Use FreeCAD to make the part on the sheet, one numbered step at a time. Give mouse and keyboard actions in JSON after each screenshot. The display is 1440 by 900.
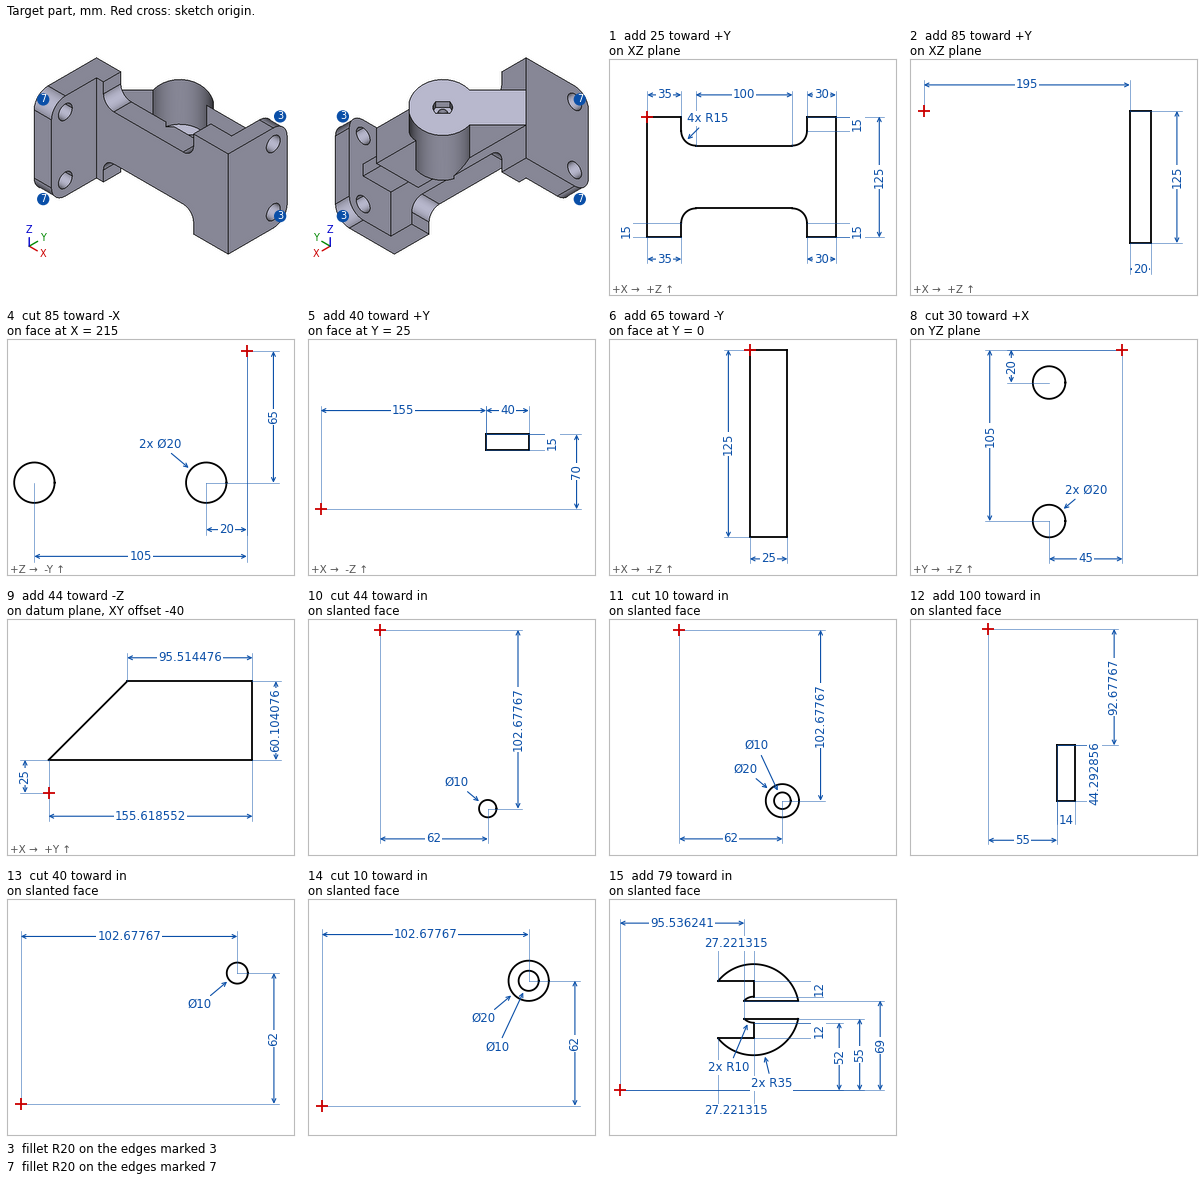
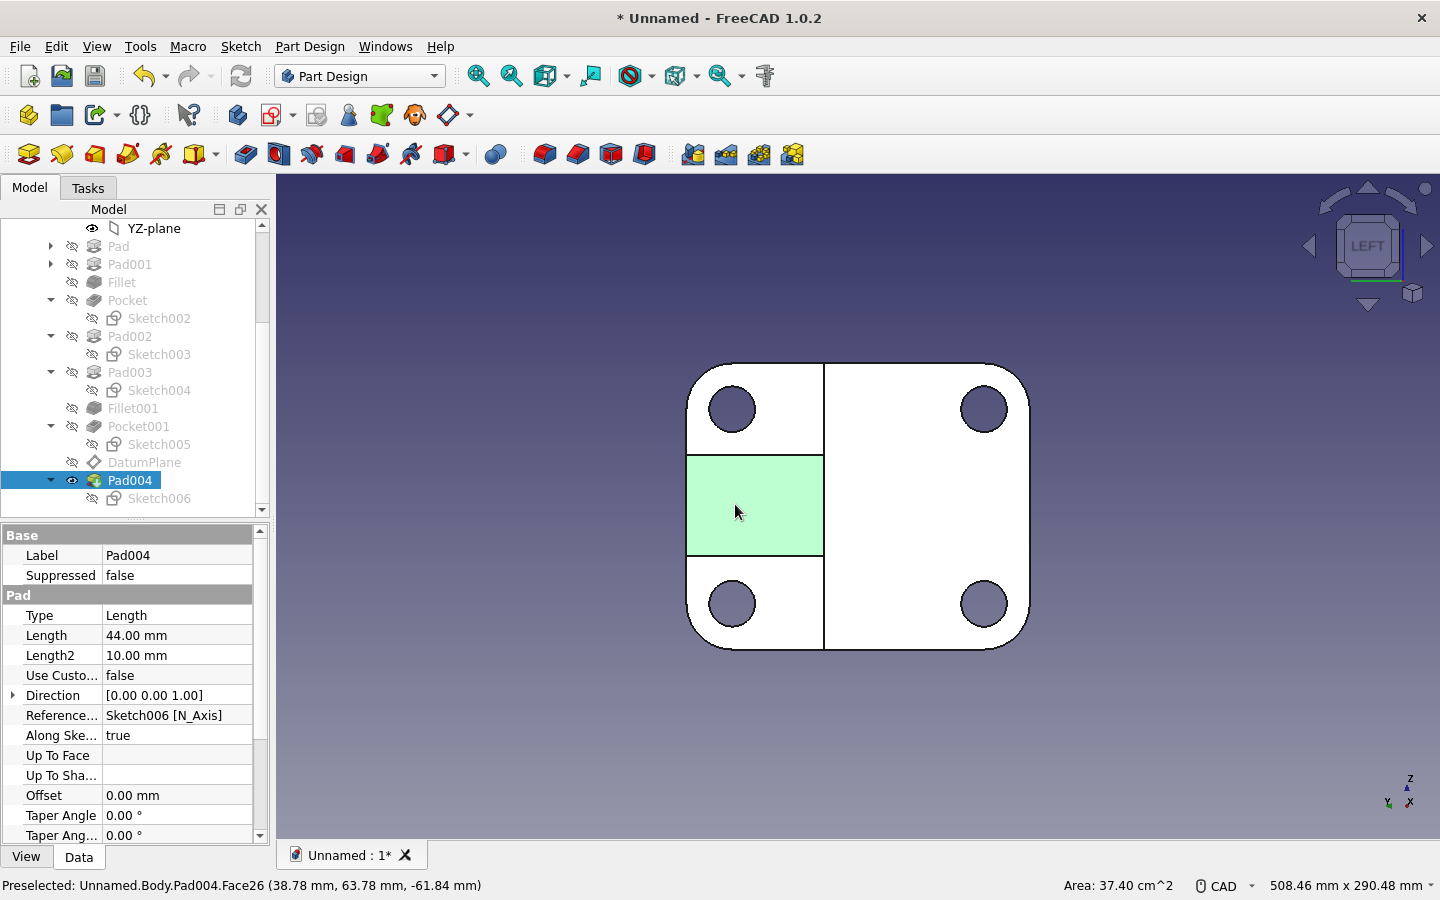
{"action": "left_click", "coordinate": [270, 116]}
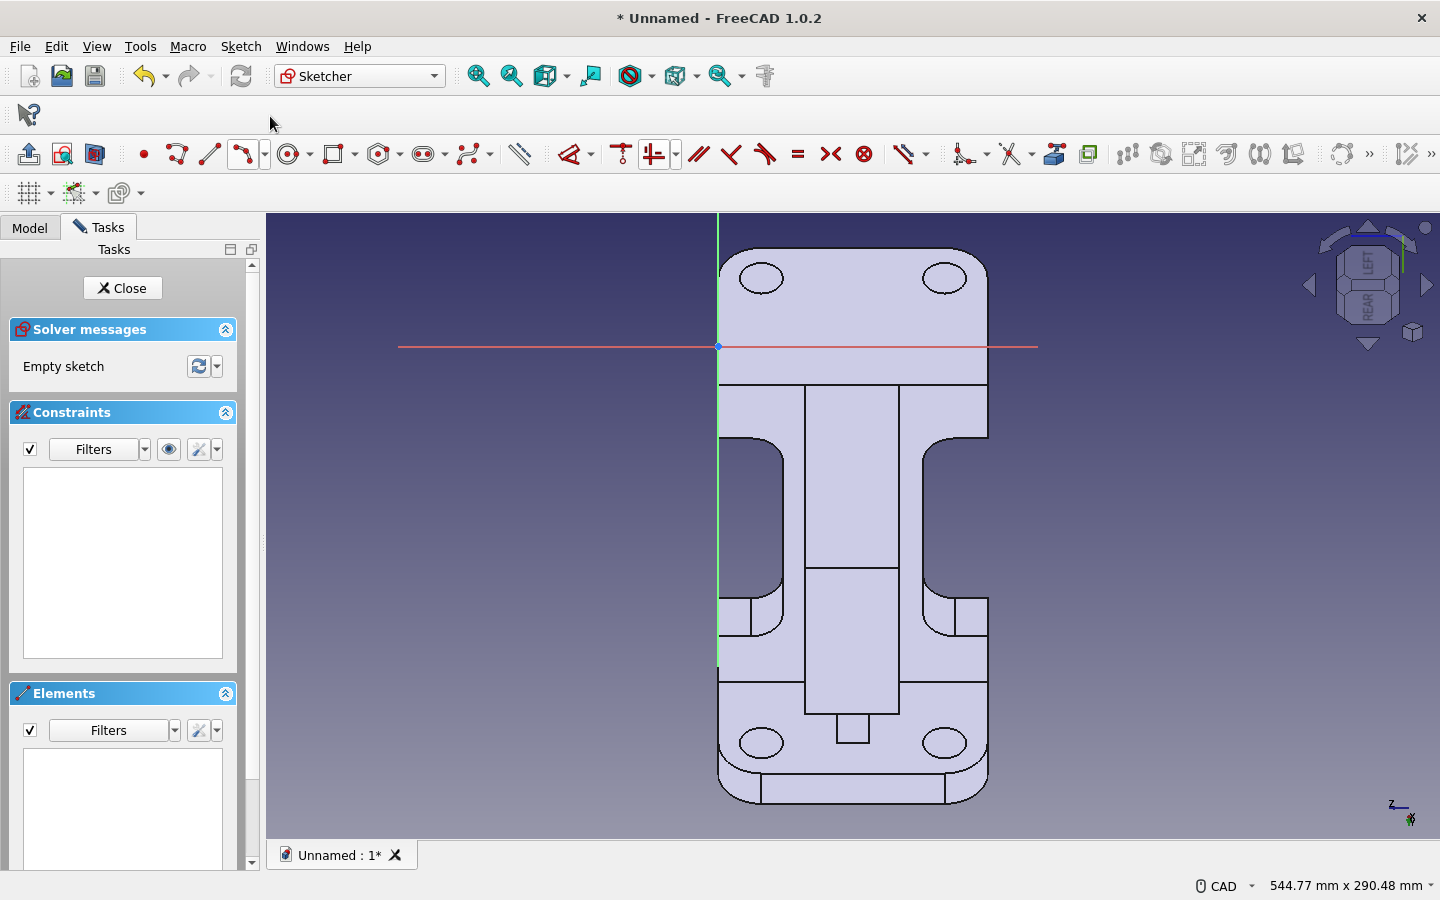
{"action": "scroll", "coordinate": [855, 570], "scroll_direction": "up", "scroll_amount": 15}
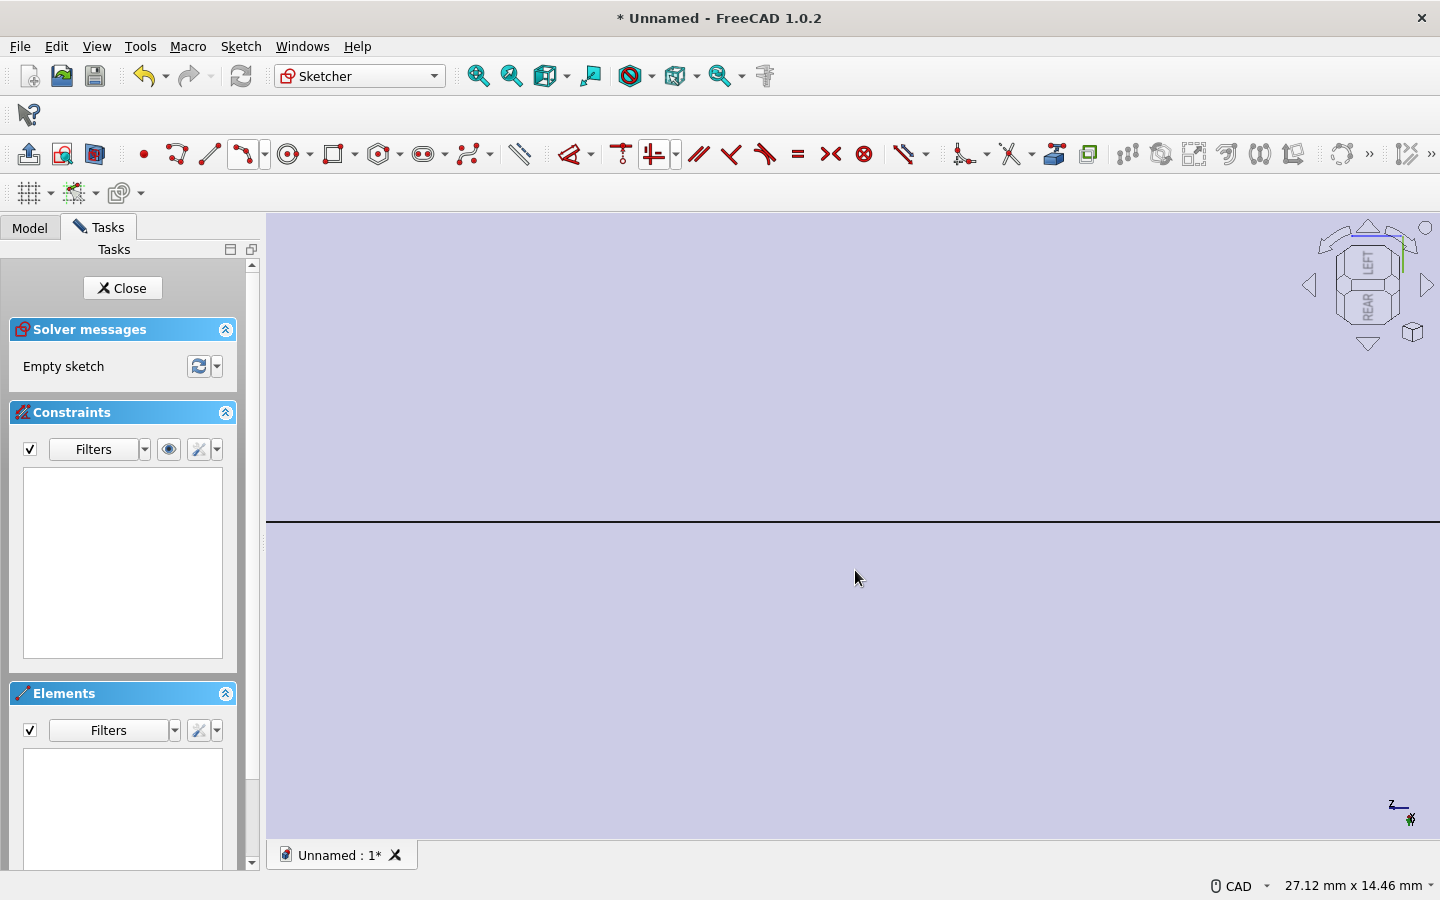
{"action": "left_click", "coordinate": [288, 154]}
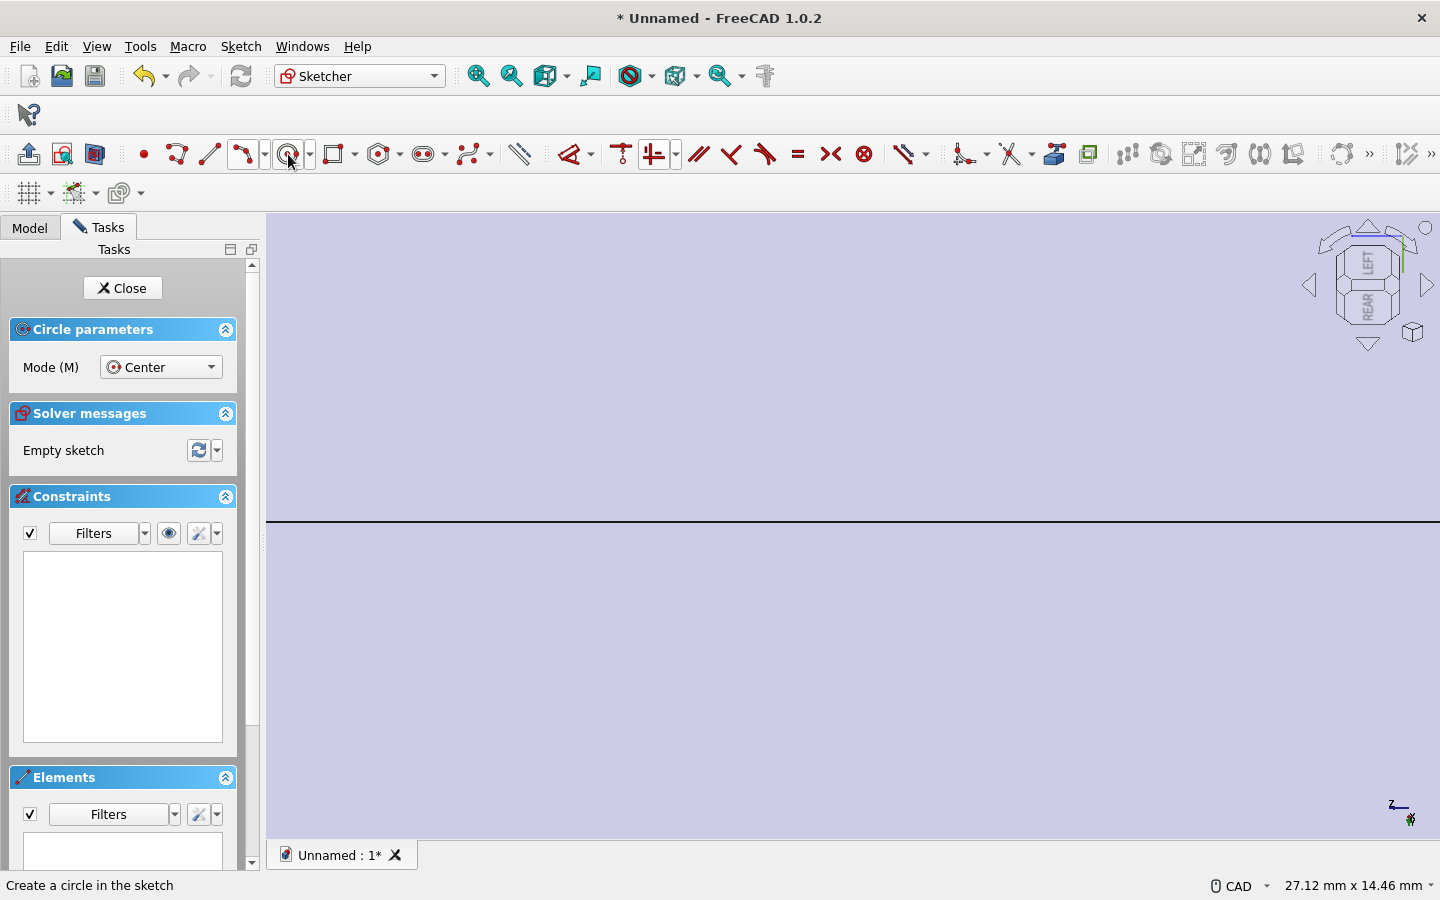
{"action": "left_click", "coordinate": [784, 522]}
{"action": "left_click", "coordinate": [937, 369]}
{"action": "key", "text": "Escape"}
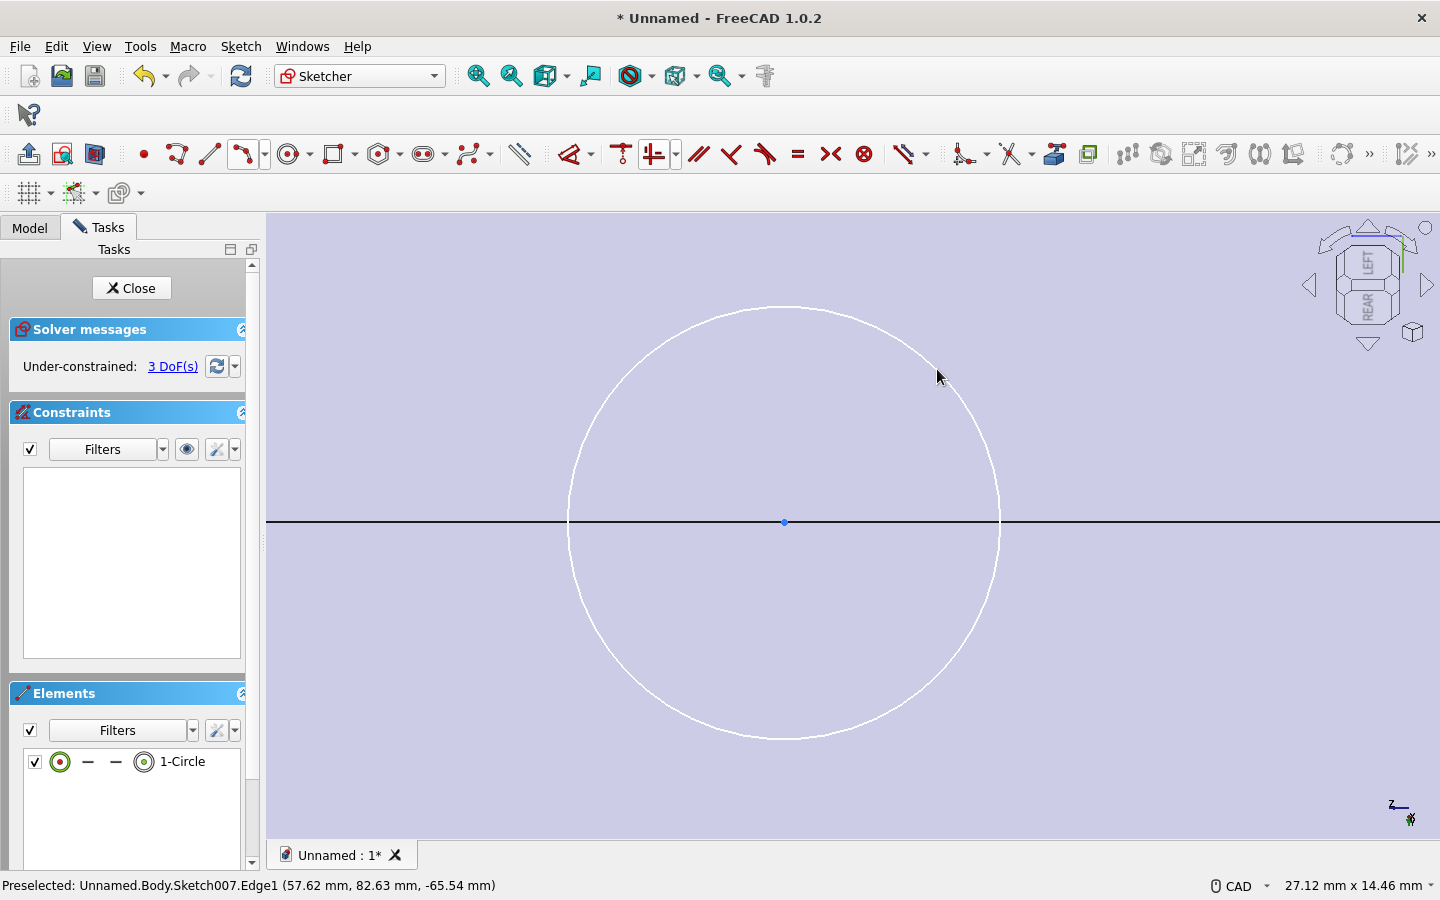
{"action": "left_click", "coordinate": [568, 154]}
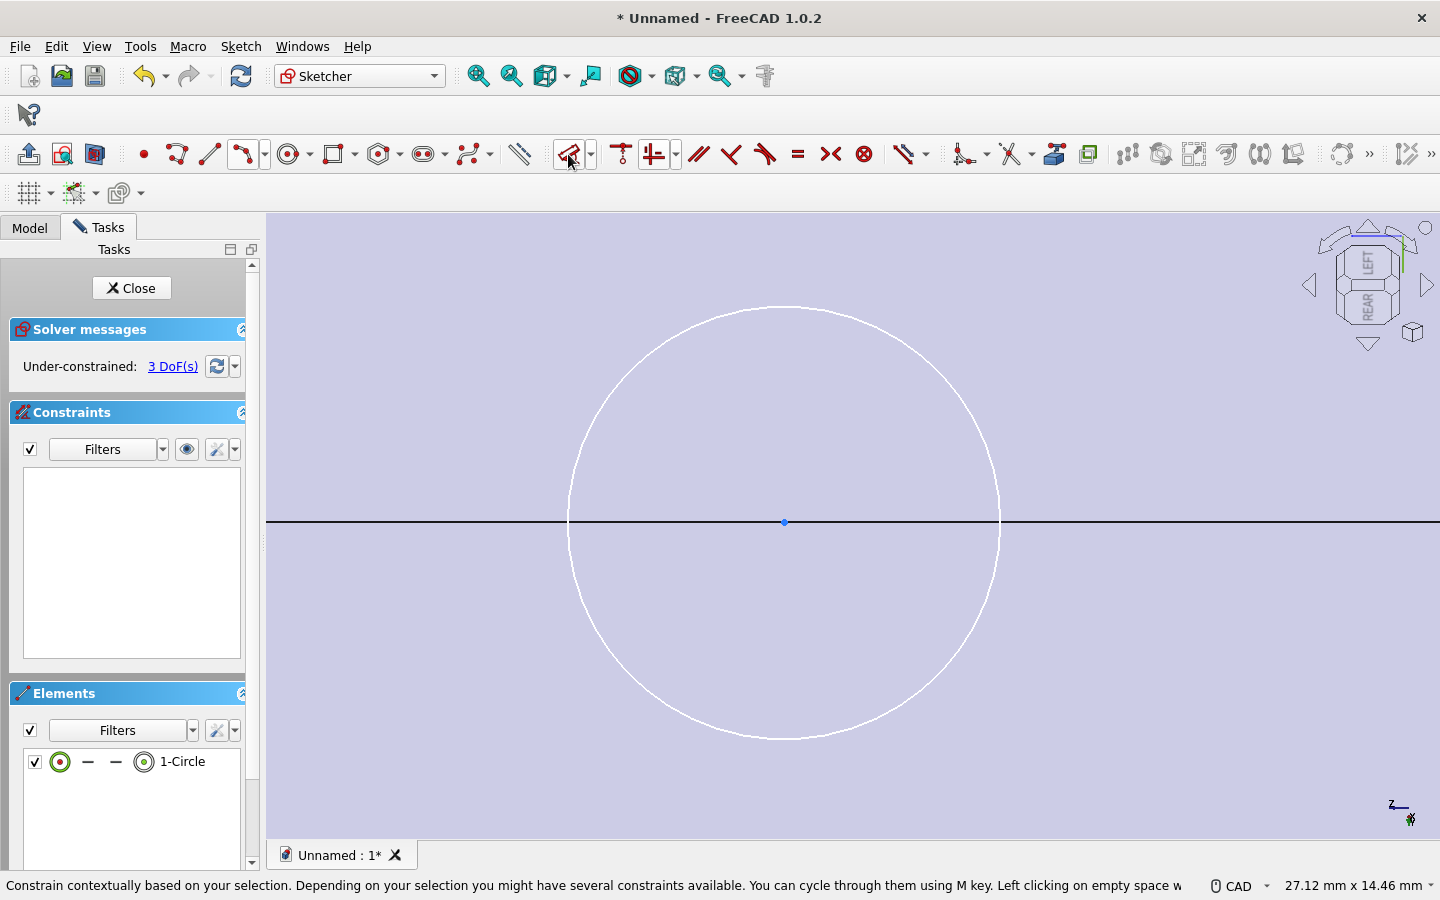
{"action": "left_click", "coordinate": [937, 370]}
{"action": "left_click", "coordinate": [960, 347]}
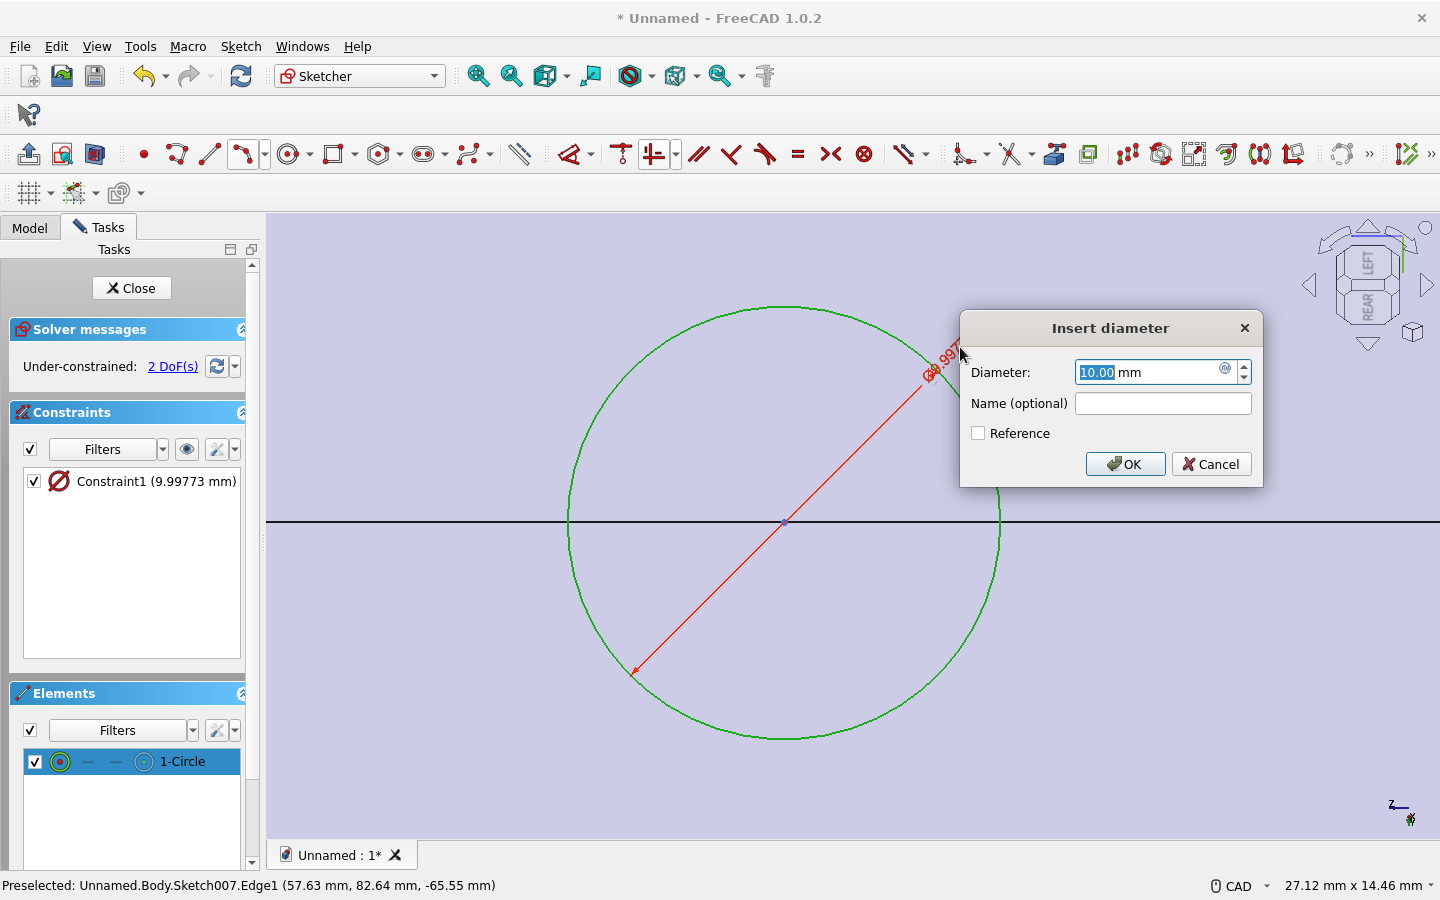
{"action": "type", "text": "10"}
{"action": "key", "text": "Return"}